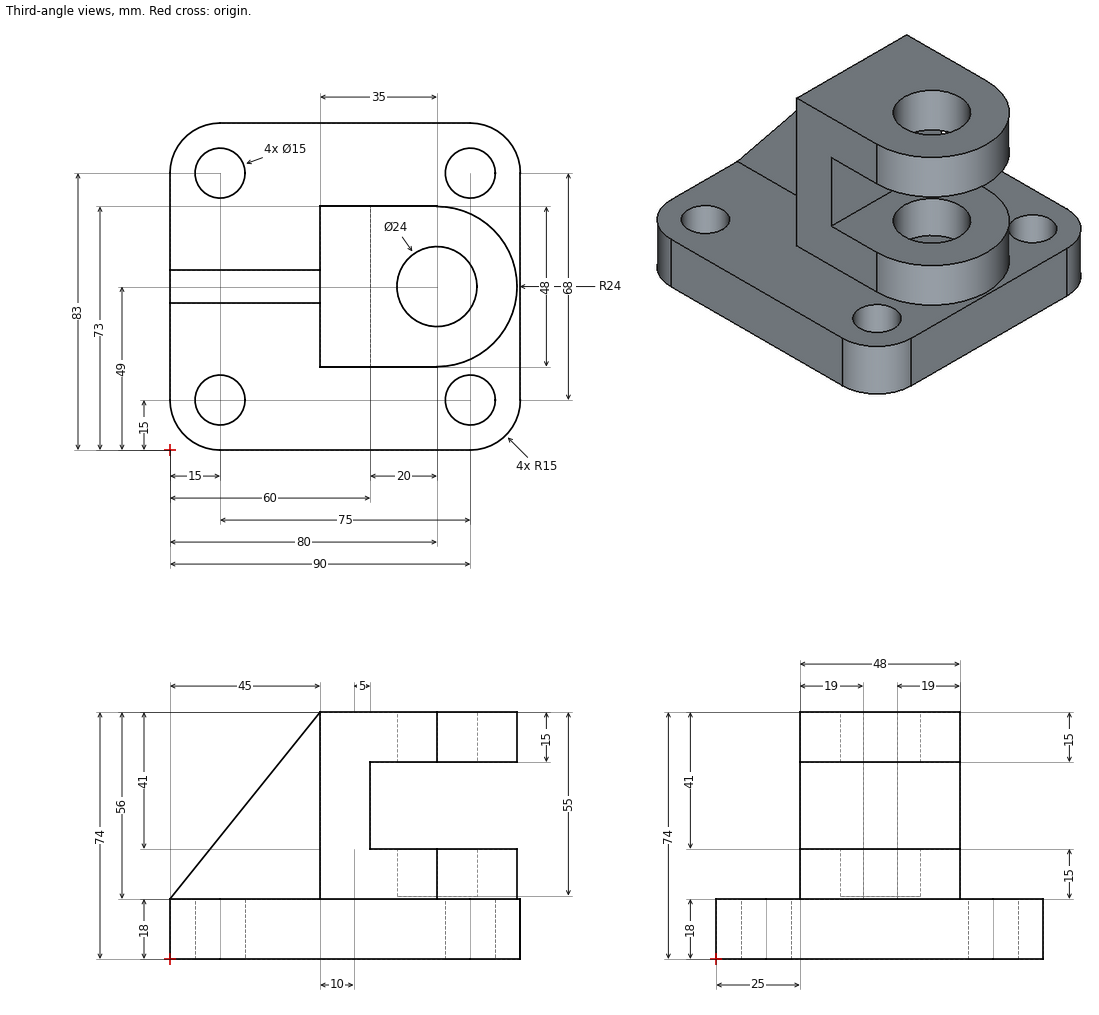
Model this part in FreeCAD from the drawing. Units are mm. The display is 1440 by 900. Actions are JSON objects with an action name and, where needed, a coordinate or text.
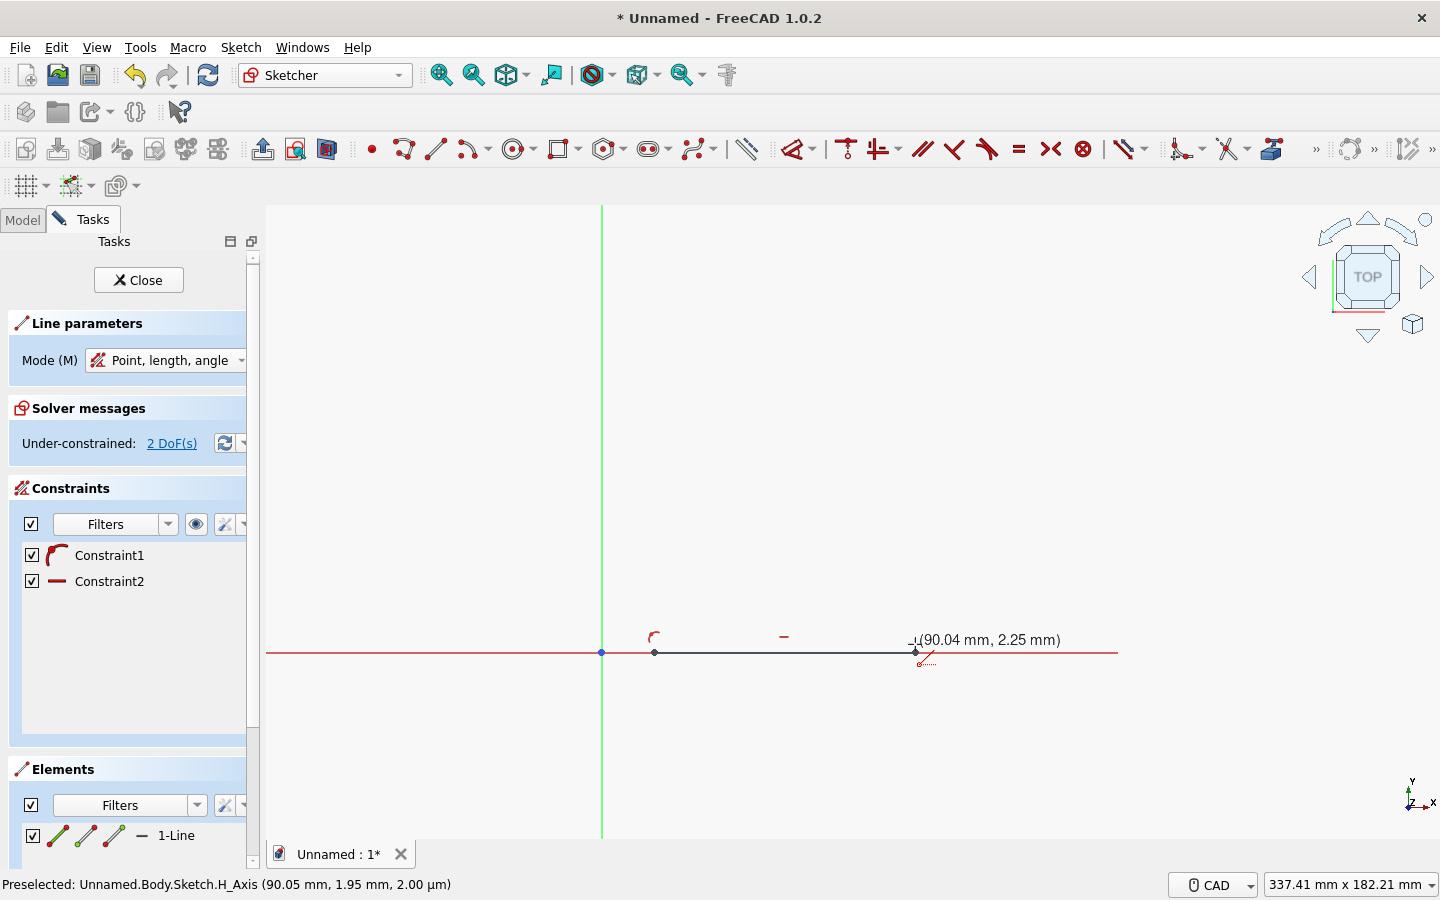
{"action": "left_click", "coordinate": [967, 601]}
{"action": "left_click", "coordinate": [967, 364]}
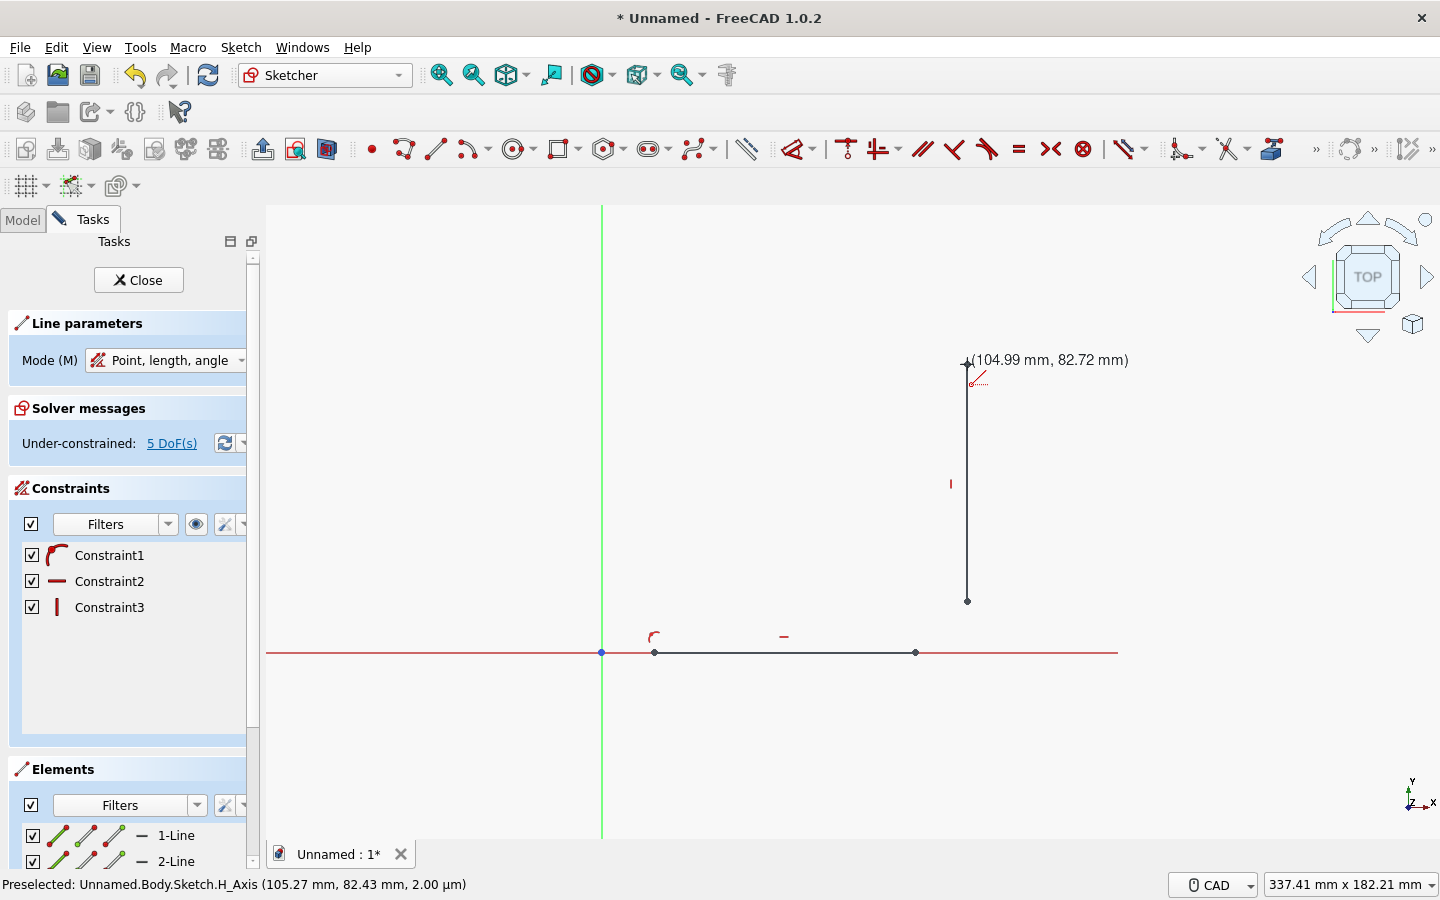
{"action": "left_click", "coordinate": [915, 312]}
{"action": "left_click", "coordinate": [654, 312]}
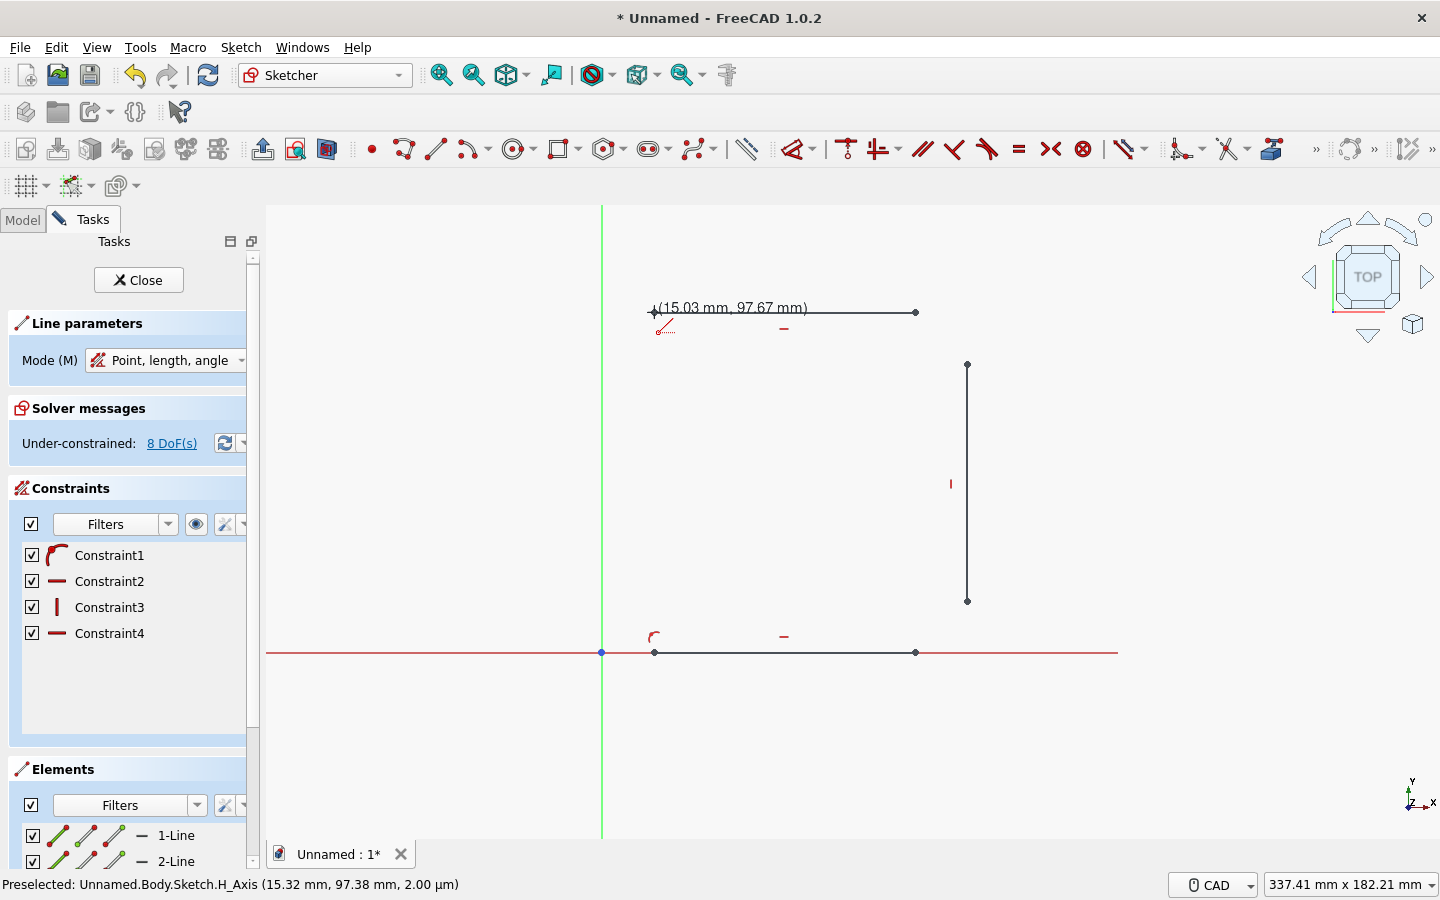
{"action": "left_click", "coordinate": [602, 364]}
{"action": "left_click", "coordinate": [611, 601]}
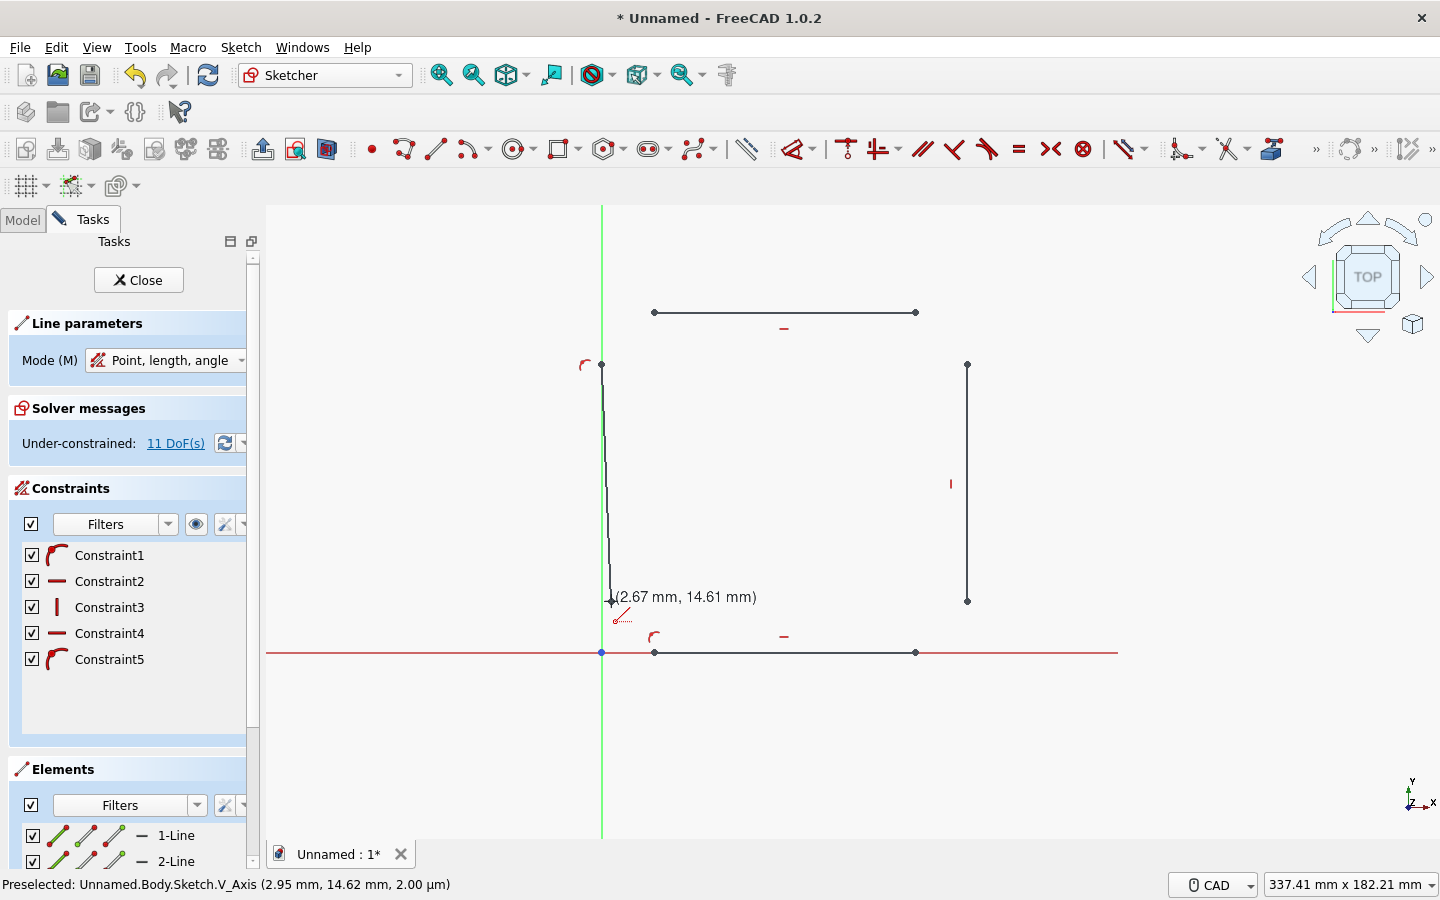
{"action": "left_click", "coordinate": [490, 150]}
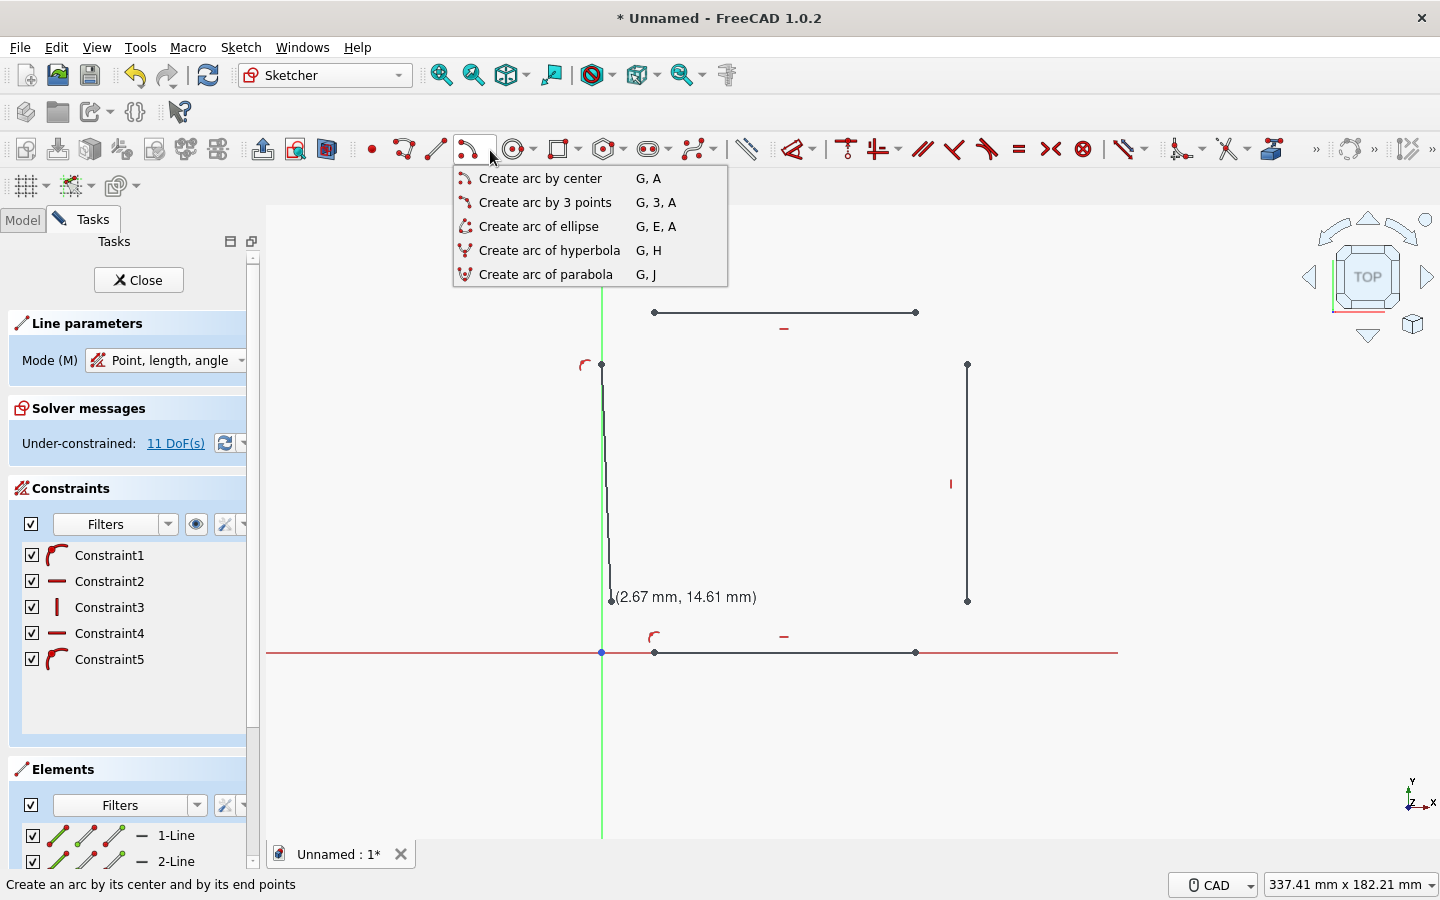
{"action": "left_click", "coordinate": [590, 202]}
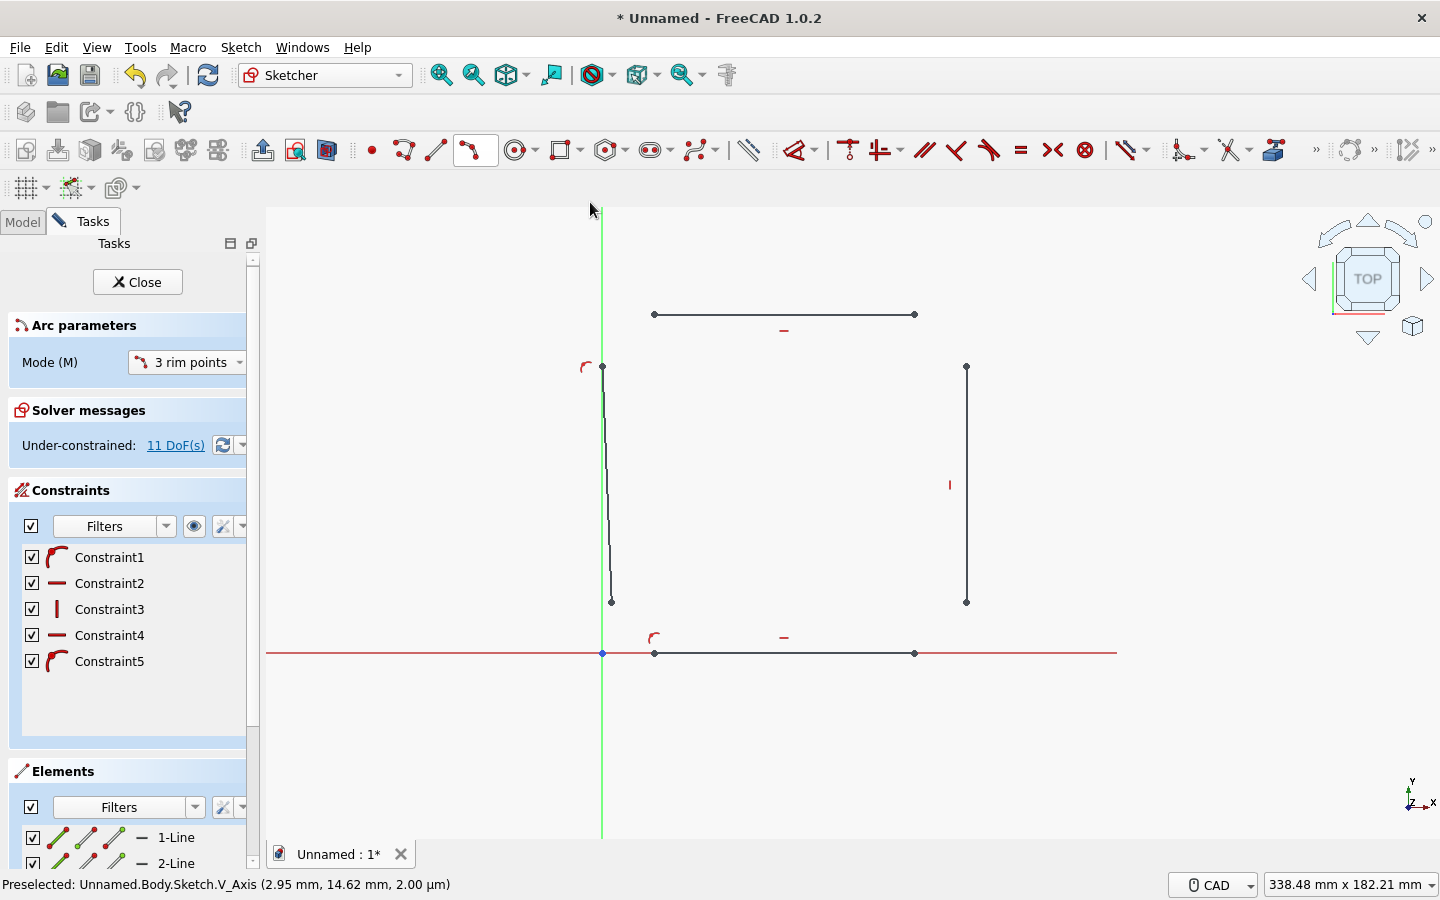
{"action": "left_click", "coordinate": [915, 653]}
{"action": "left_click", "coordinate": [967, 603]}
{"action": "left_click", "coordinate": [951, 638]}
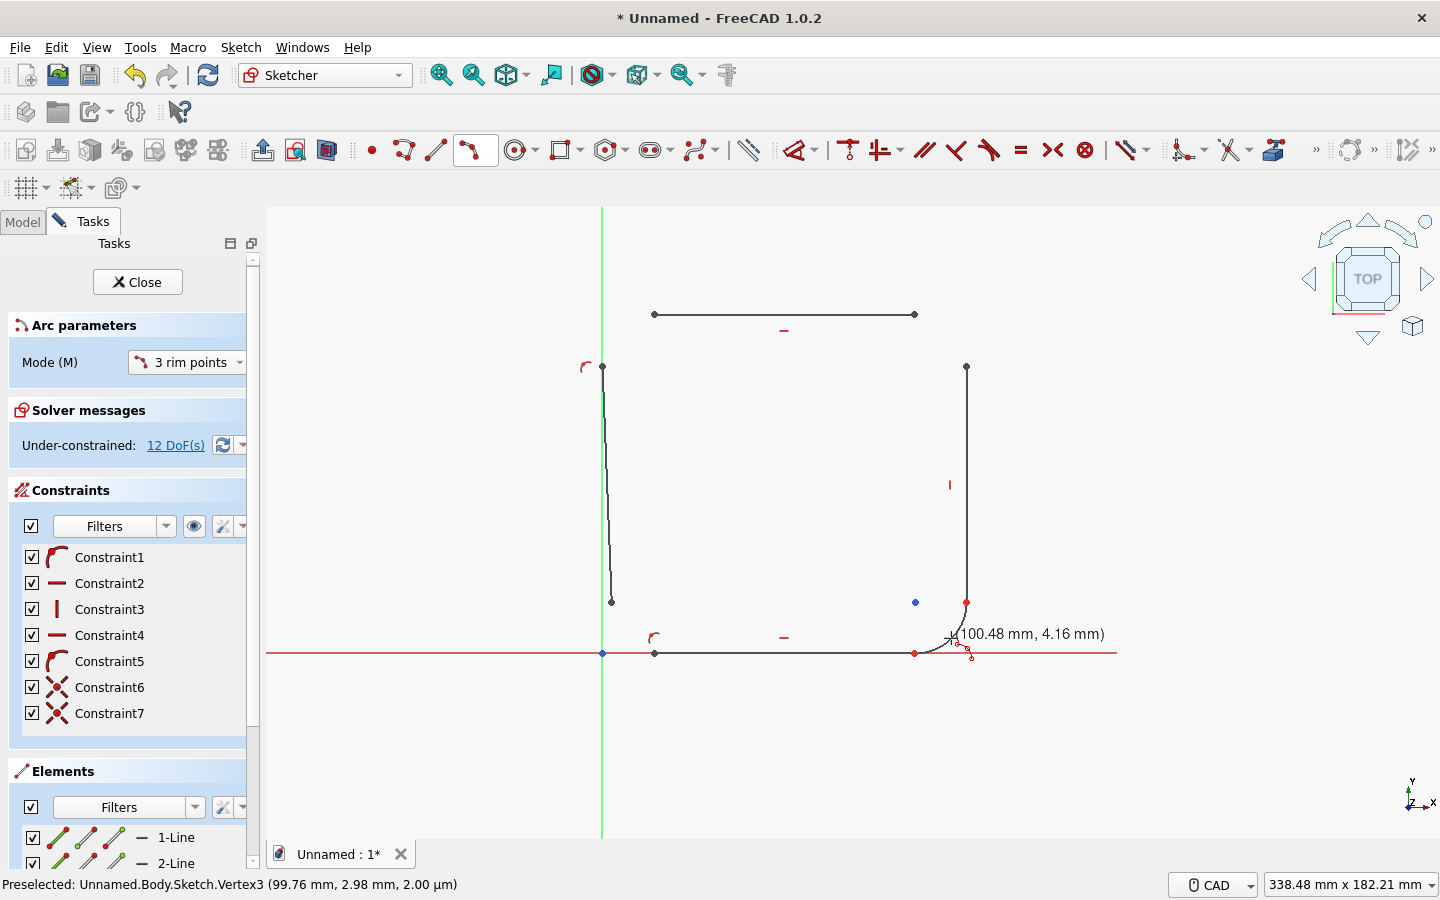
{"action": "left_click", "coordinate": [967, 366]}
{"action": "left_click", "coordinate": [915, 315]}
{"action": "left_click", "coordinate": [951, 329]}